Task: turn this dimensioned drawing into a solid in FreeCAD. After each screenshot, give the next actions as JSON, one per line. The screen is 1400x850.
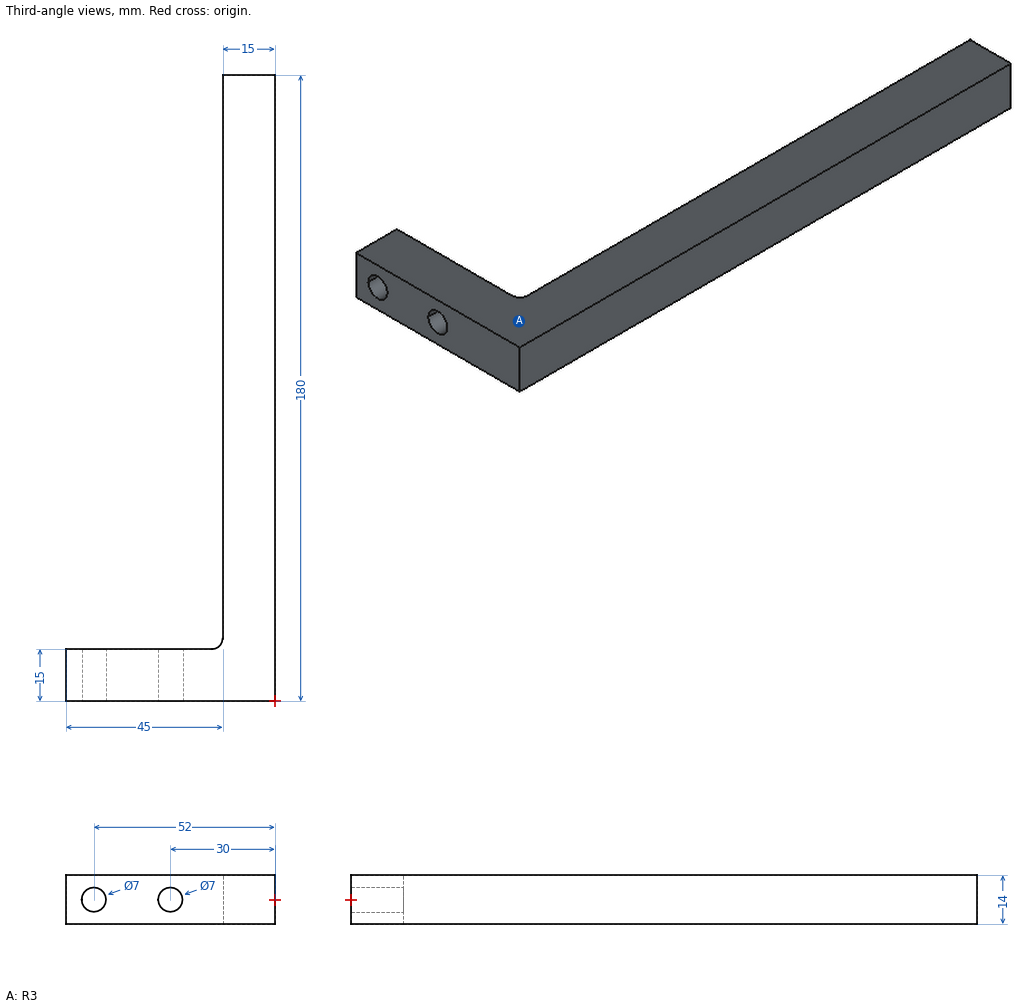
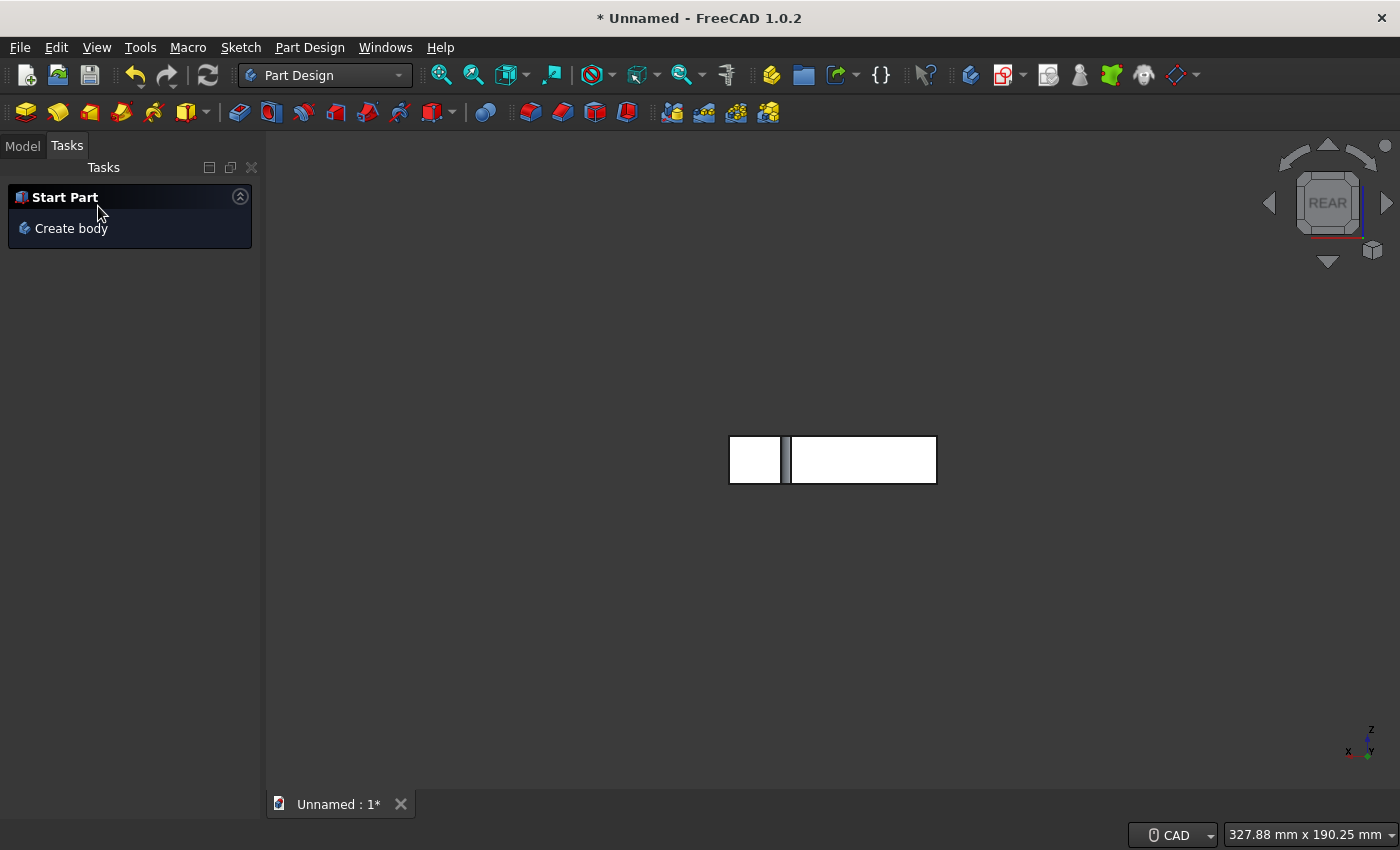
{"action": "left_click", "coordinate": [442, 76]}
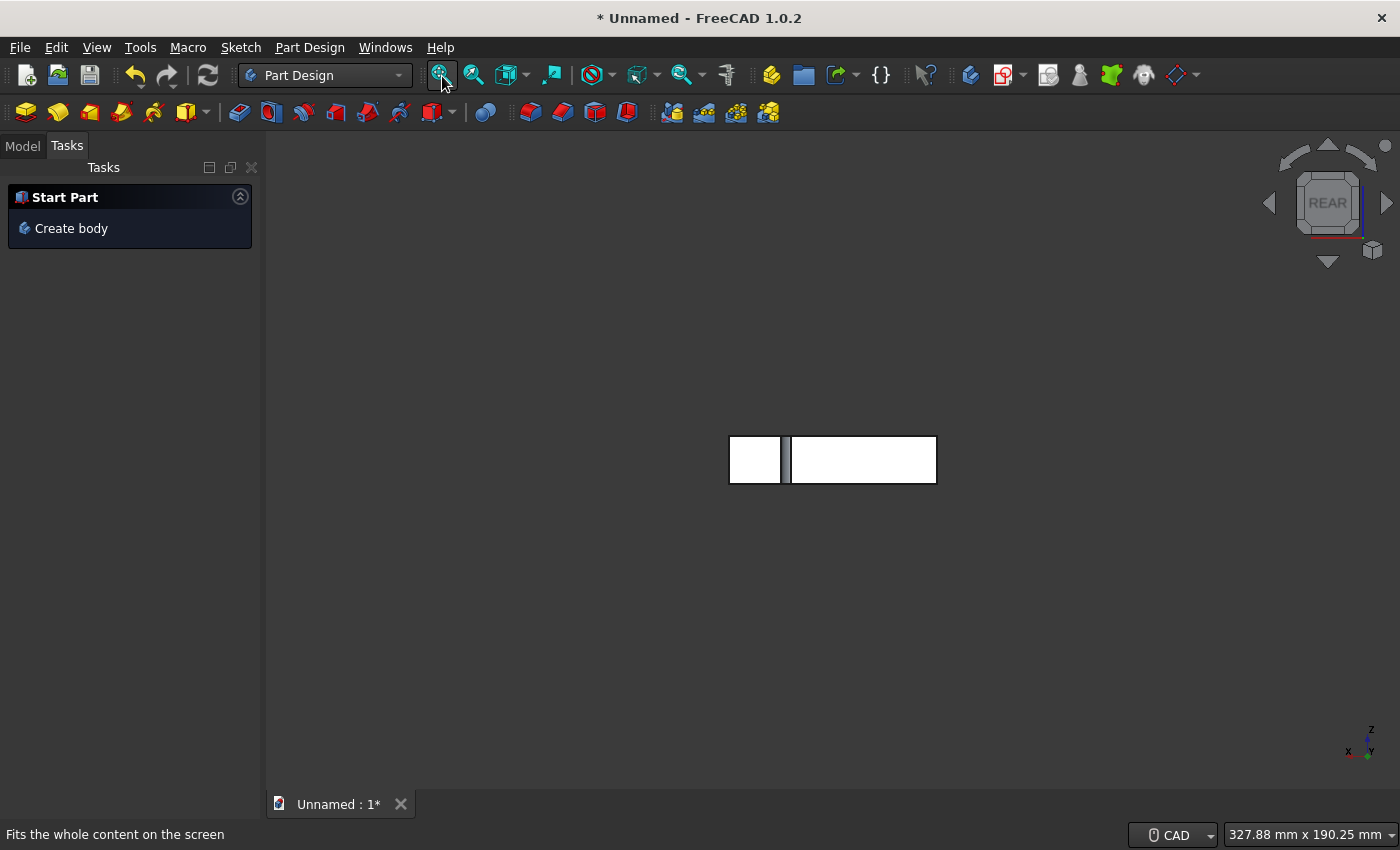
{"action": "left_click", "coordinate": [823, 459]}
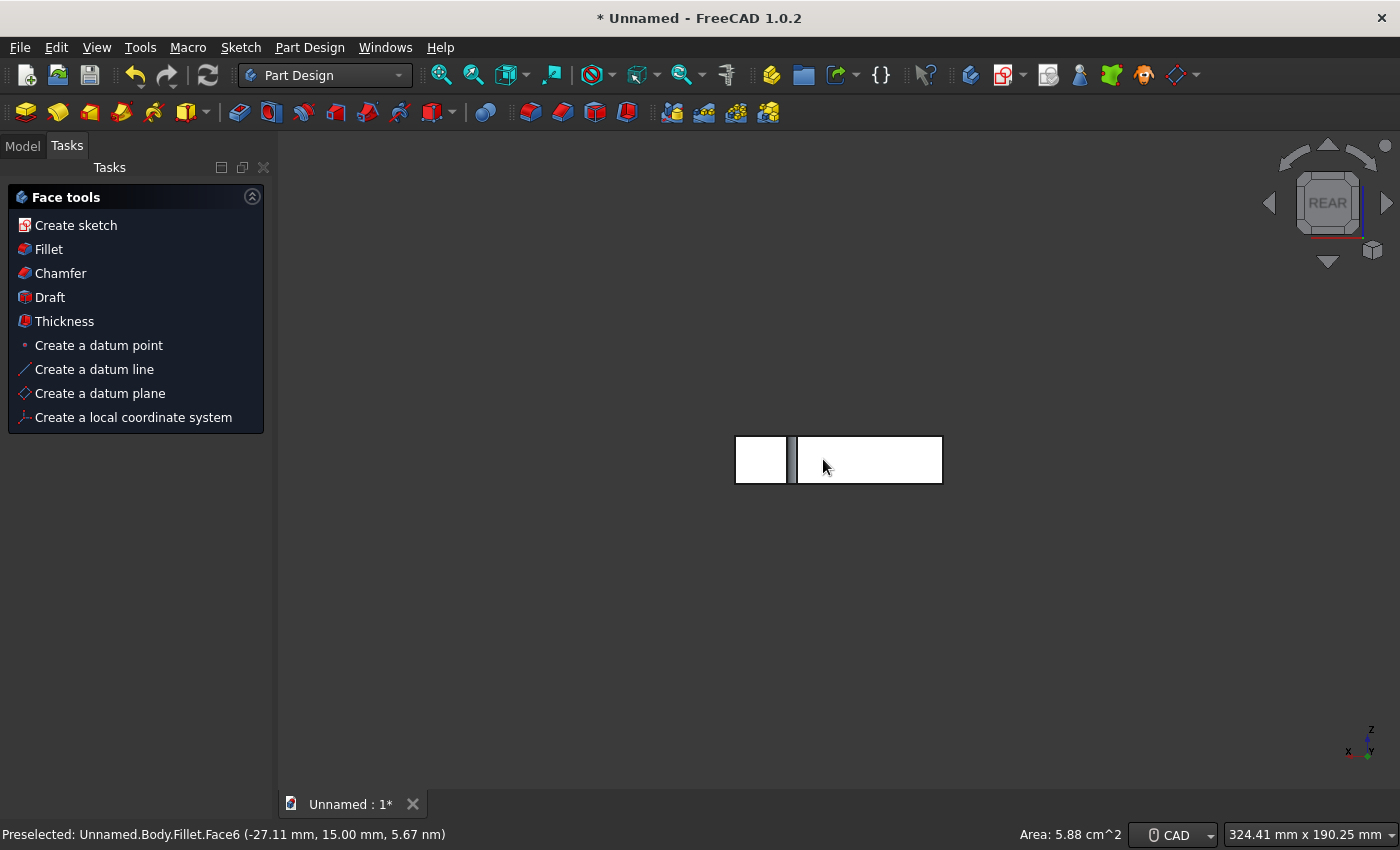
{"action": "left_click", "coordinate": [1004, 76]}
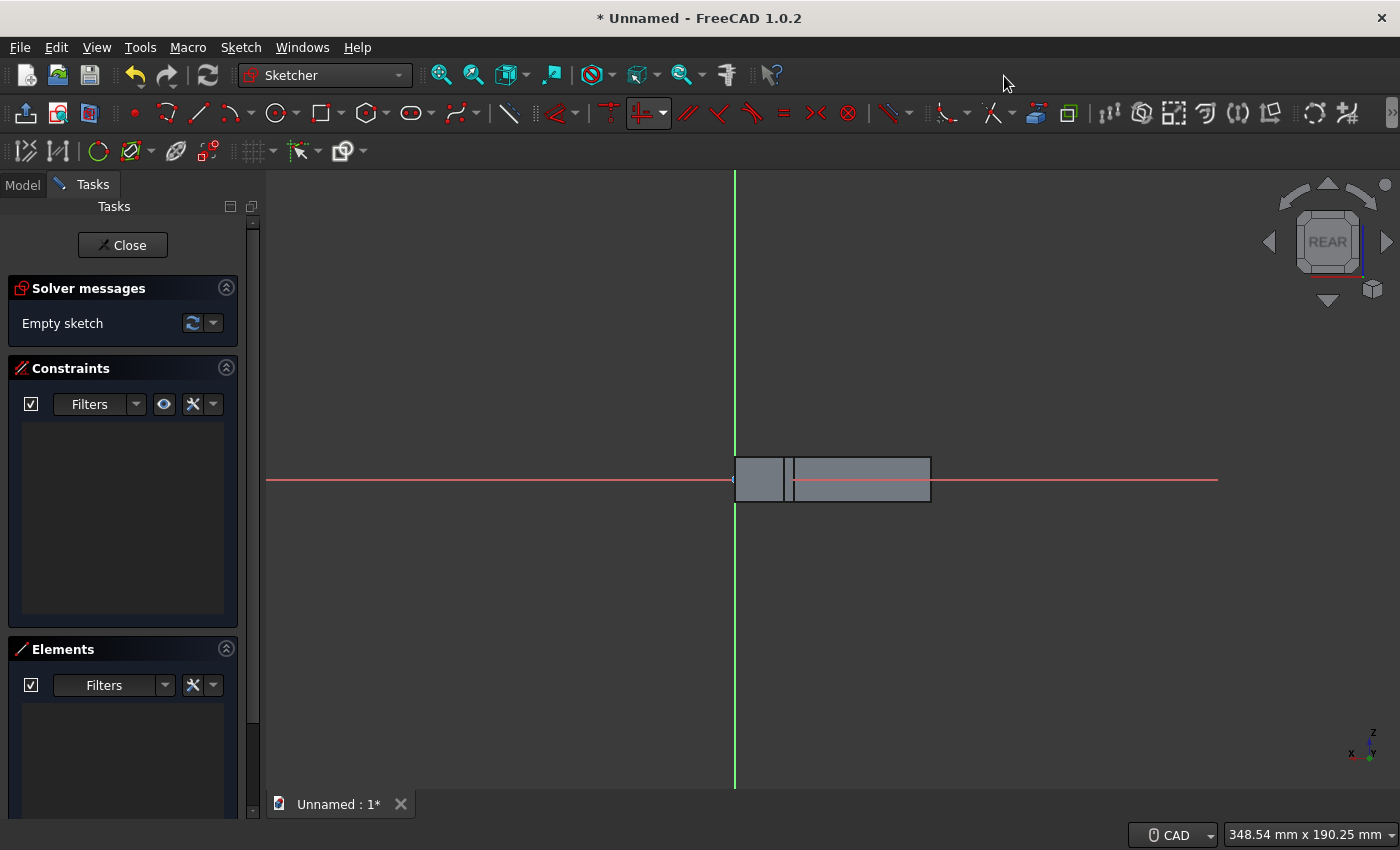
{"action": "left_click", "coordinate": [90, 114]}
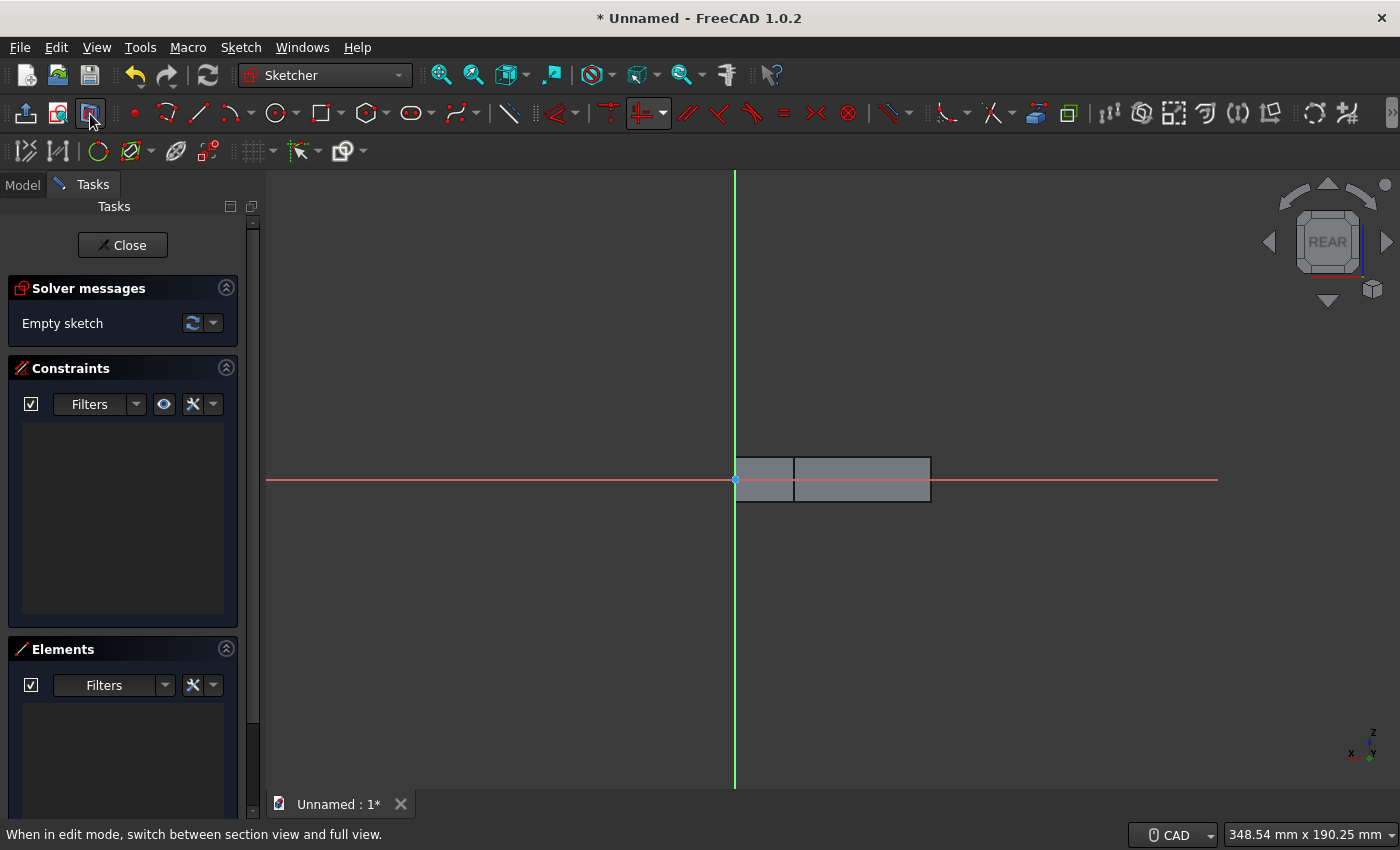
{"action": "scroll", "coordinate": [914, 480], "scroll_direction": "up", "scroll_amount": 14}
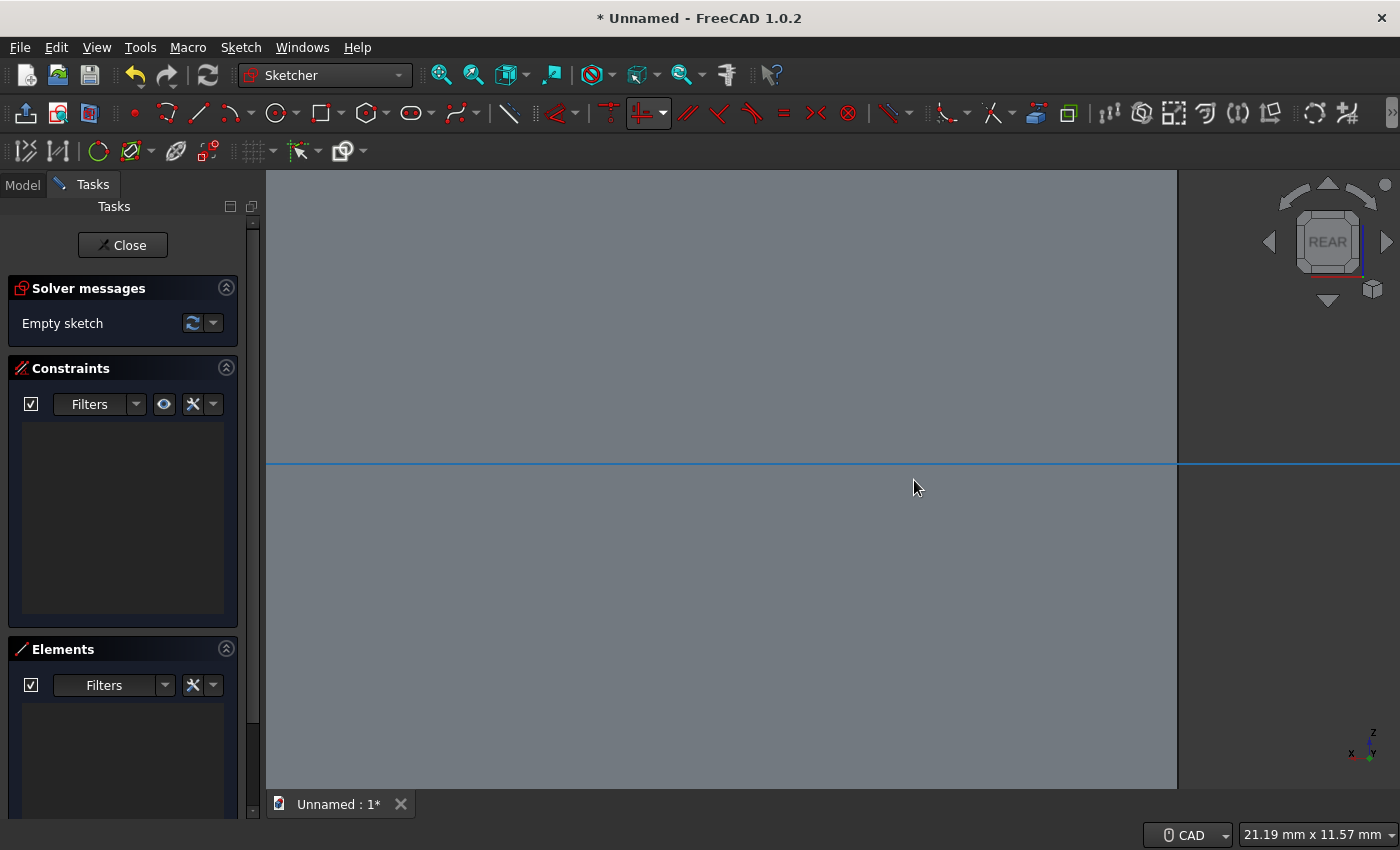
{"action": "left_click", "coordinate": [276, 114]}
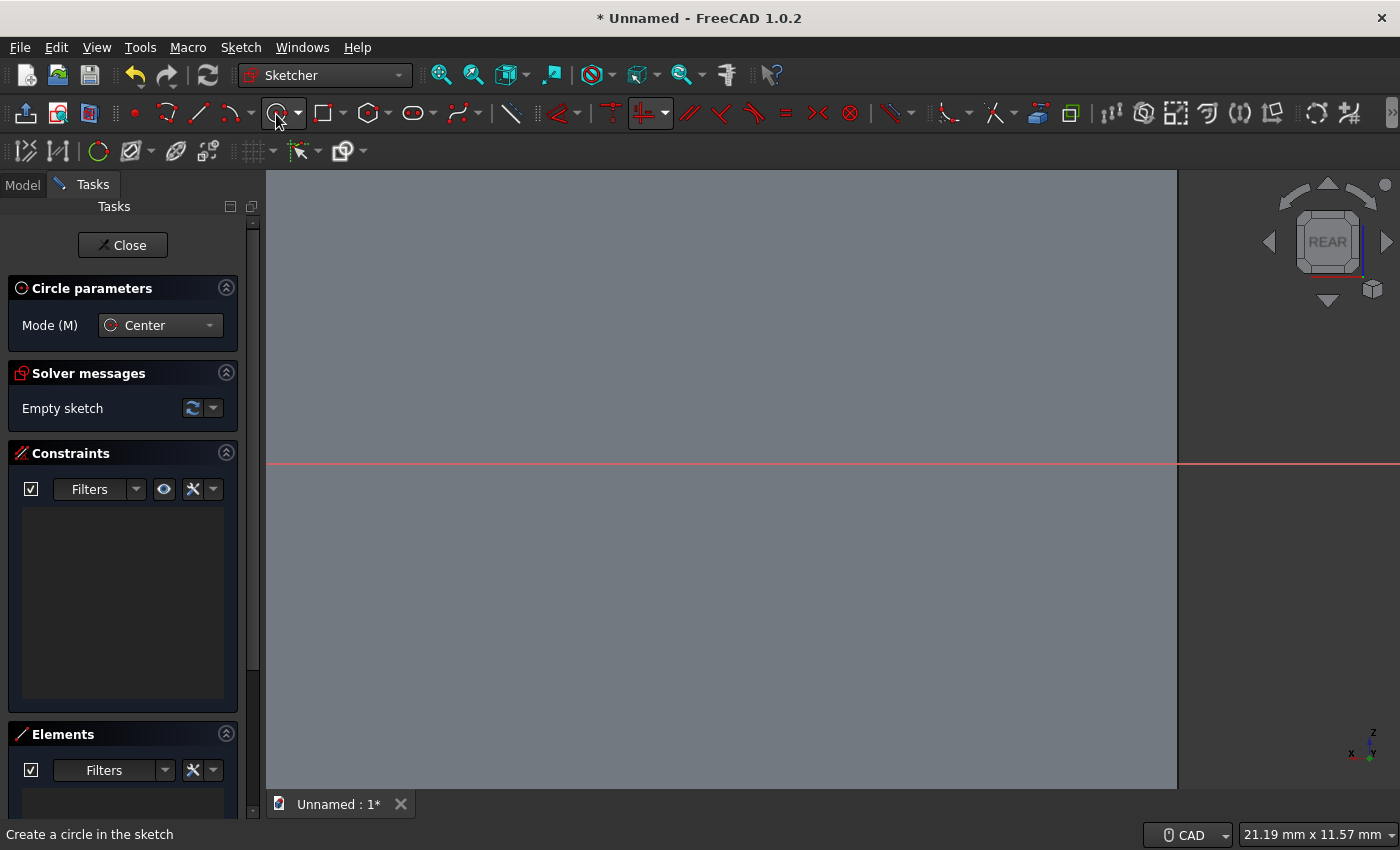
{"action": "left_click", "coordinate": [750, 464]}
{"action": "mouse_move", "coordinate": [883, 332]}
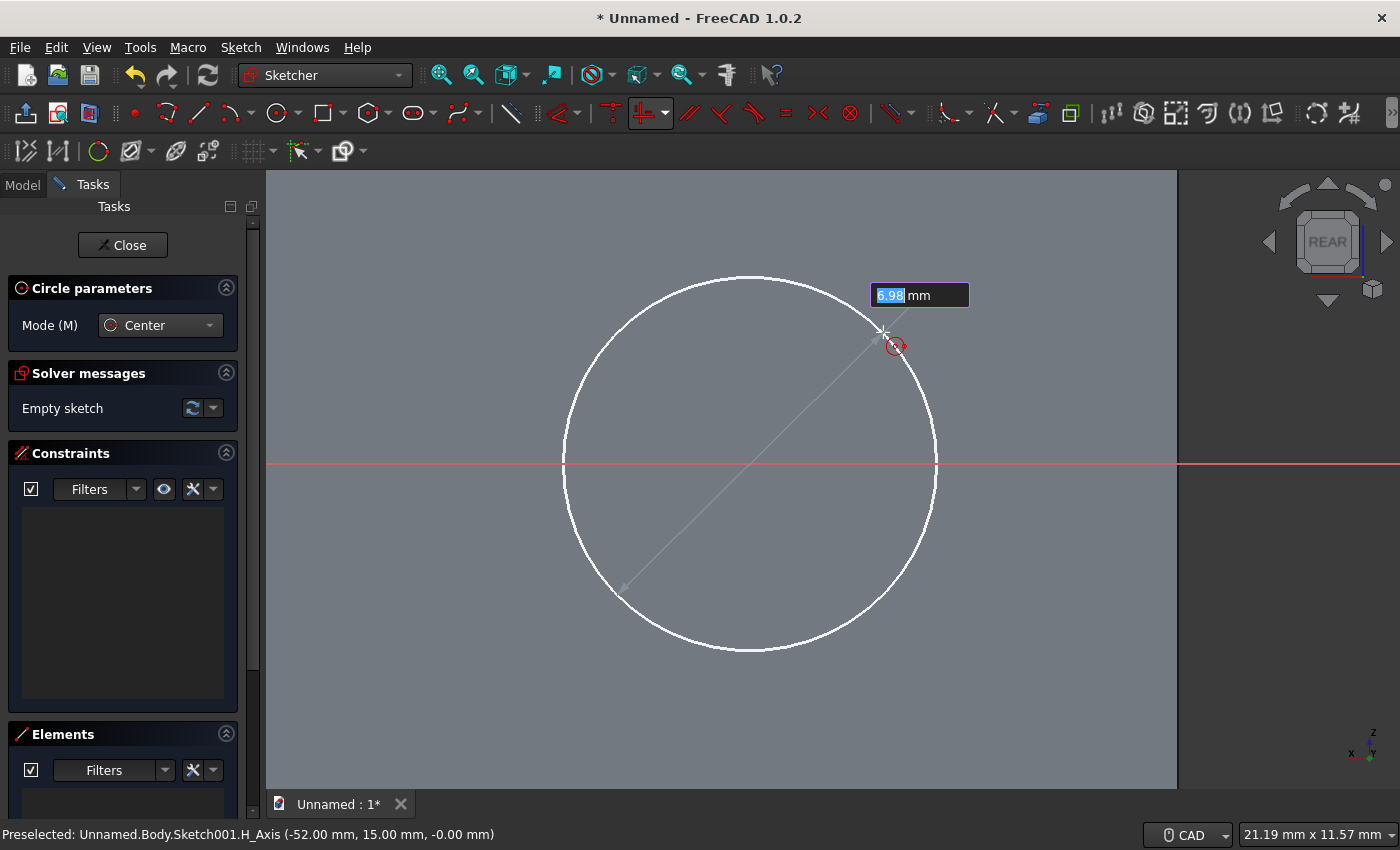
{"action": "type", "text": "7"}
{"action": "key", "text": "Return"}
{"action": "key", "text": "Escape"}